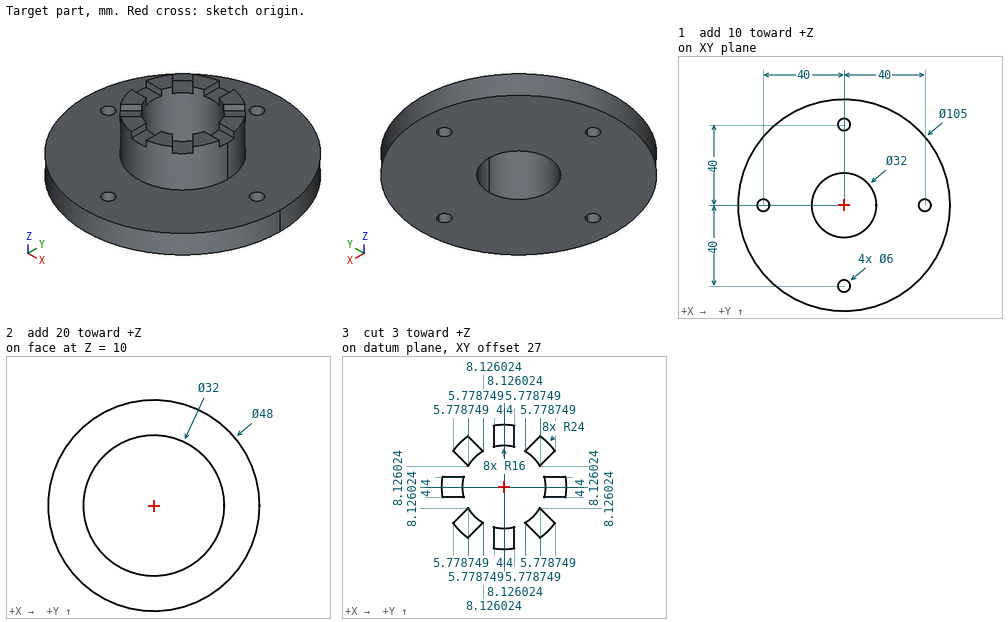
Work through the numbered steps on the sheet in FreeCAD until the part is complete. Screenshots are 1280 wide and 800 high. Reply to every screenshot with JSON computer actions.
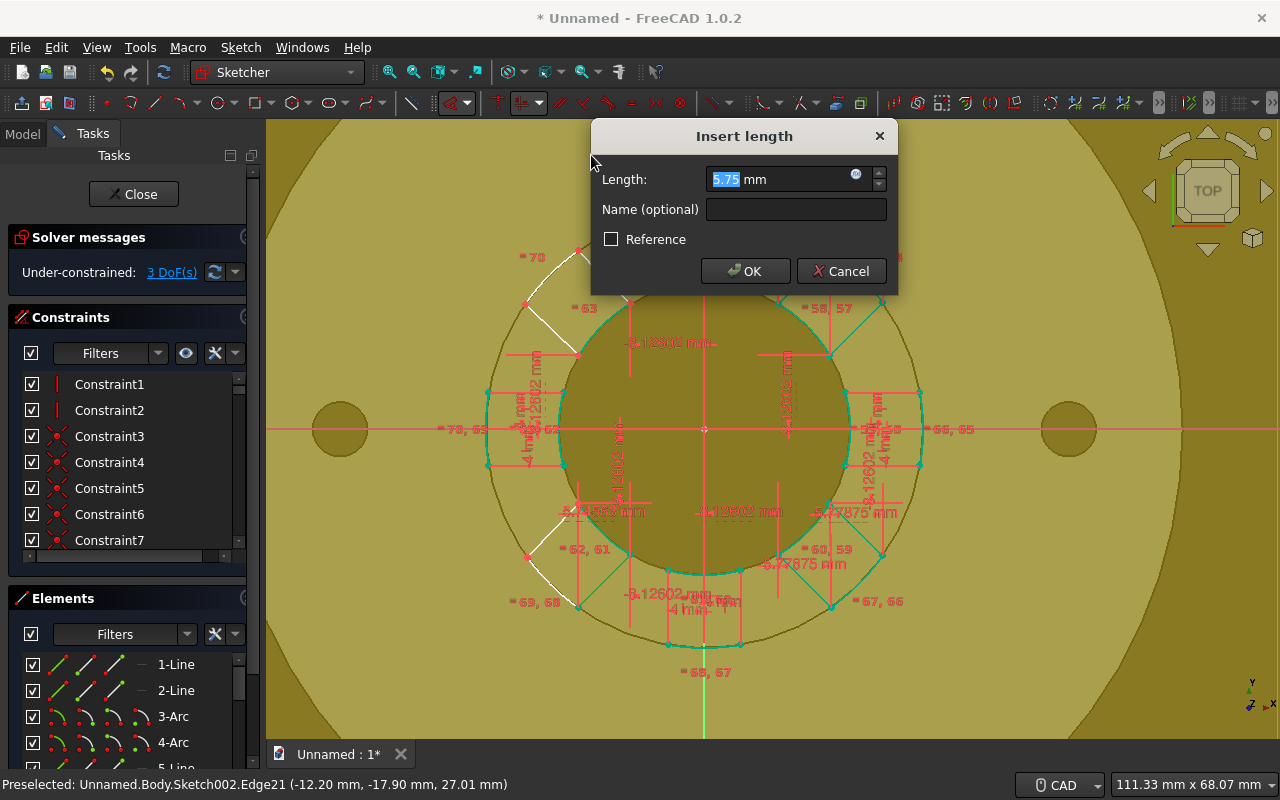
{"action": "type", "text": "5.778749"}
{"action": "key", "text": "Return"}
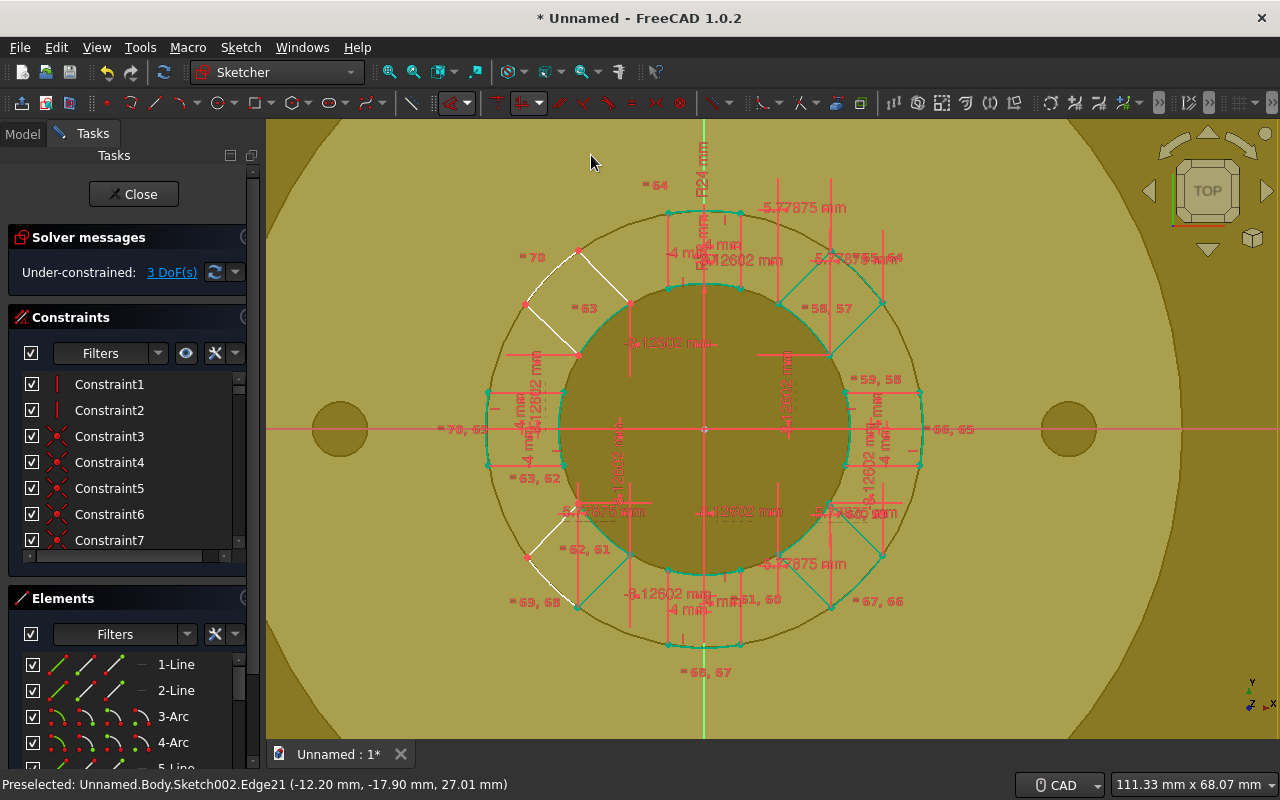
{"action": "left_click", "coordinate": [543, 541]}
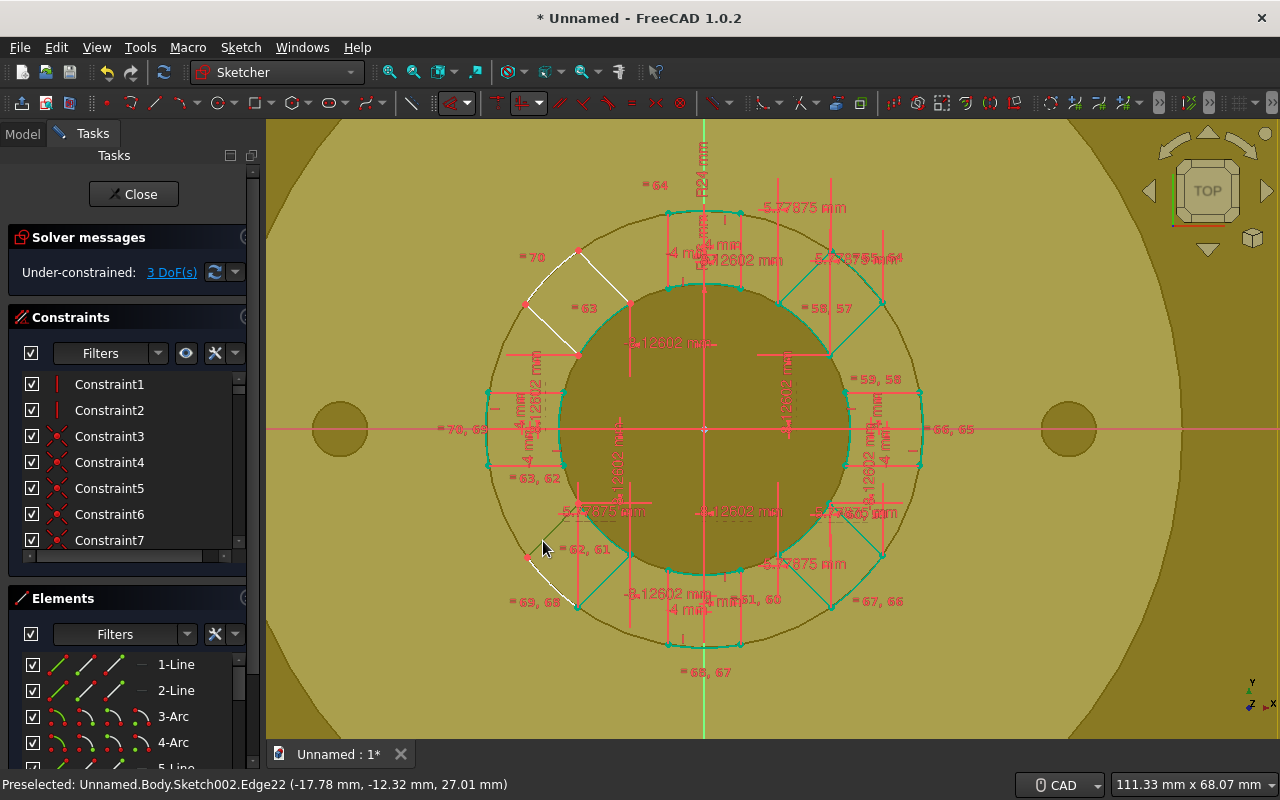
{"action": "left_click", "coordinate": [470, 104]}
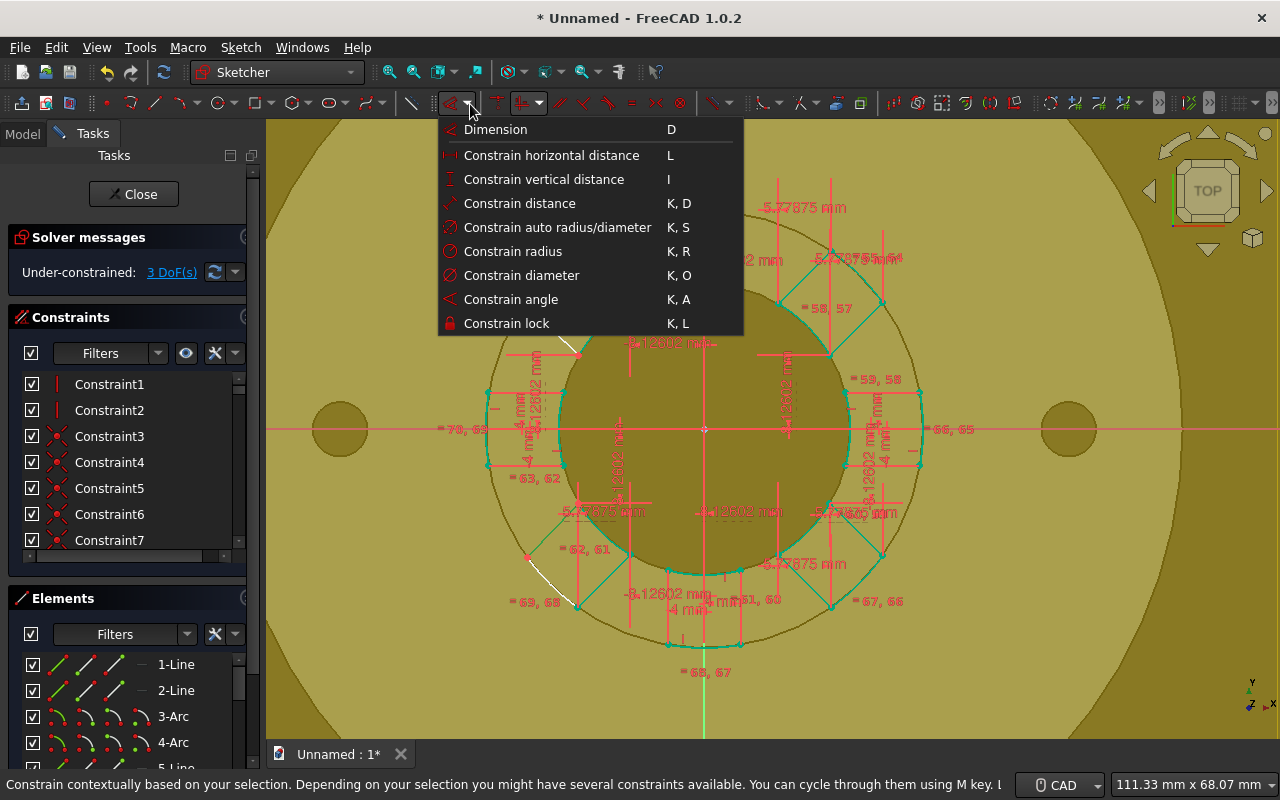
{"action": "left_click", "coordinate": [591, 155]}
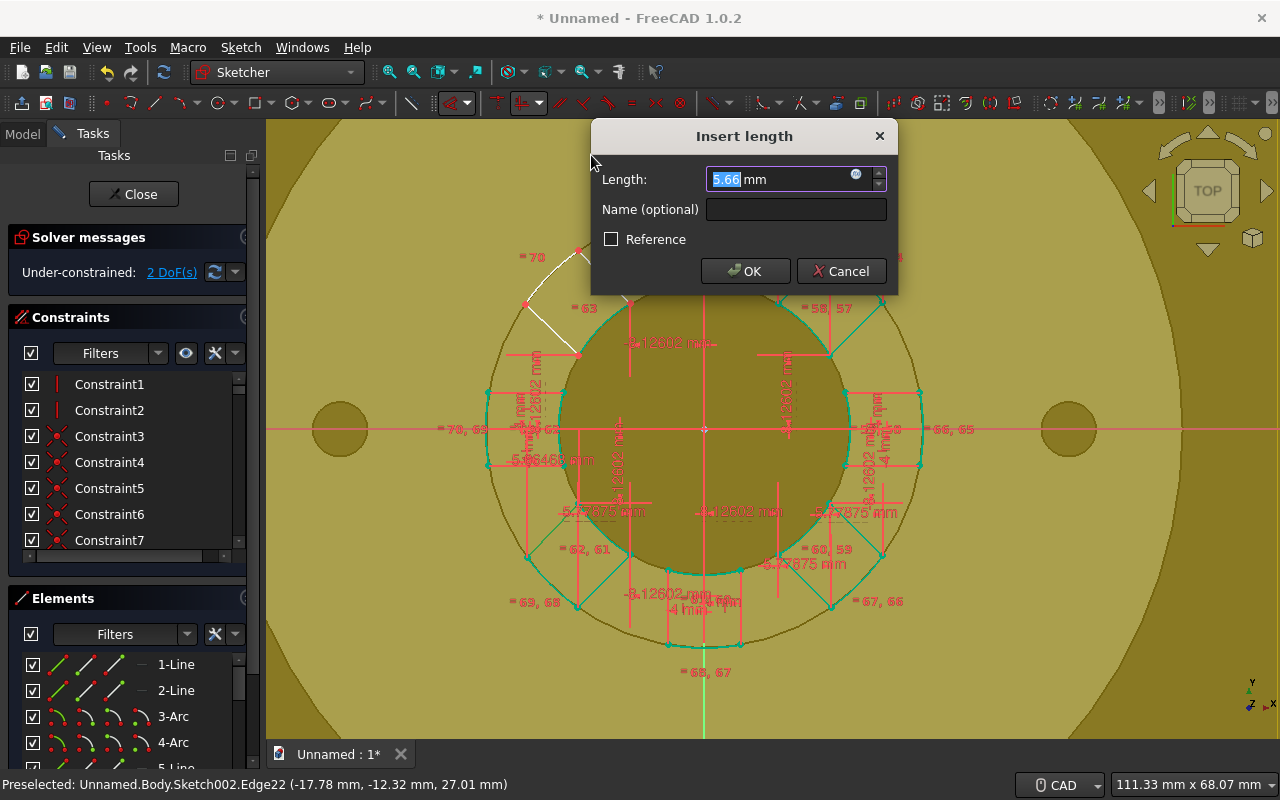
{"action": "type", "text": "5.778749"}
{"action": "key", "text": "Return"}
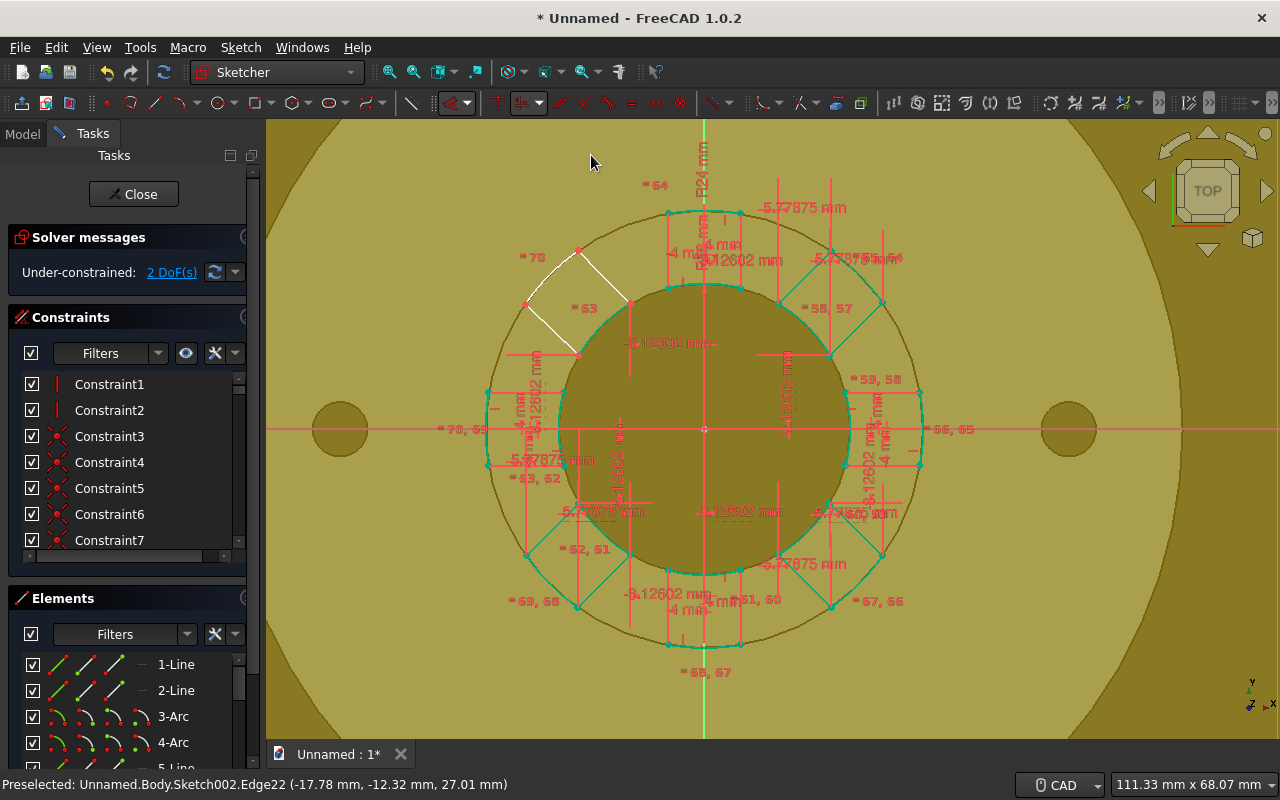
{"action": "left_click", "coordinate": [541, 319]}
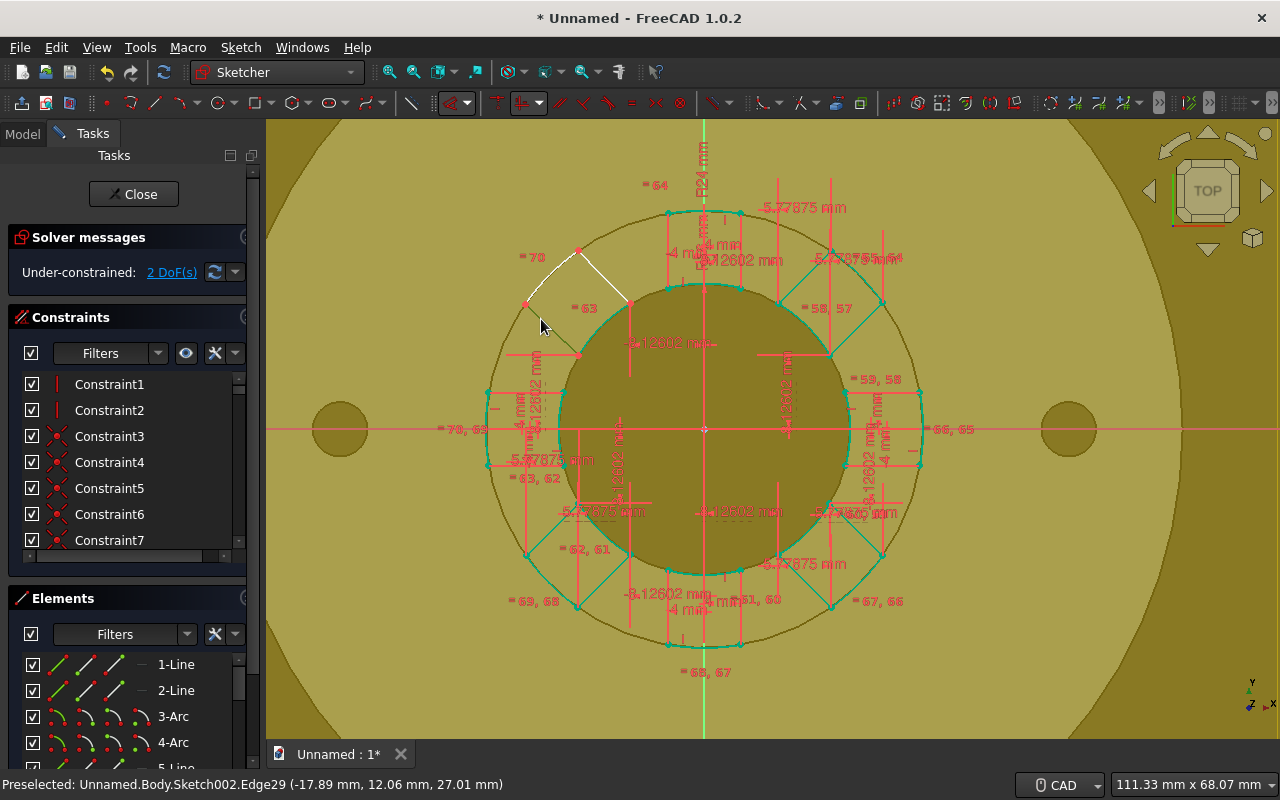
{"action": "left_click", "coordinate": [470, 104]}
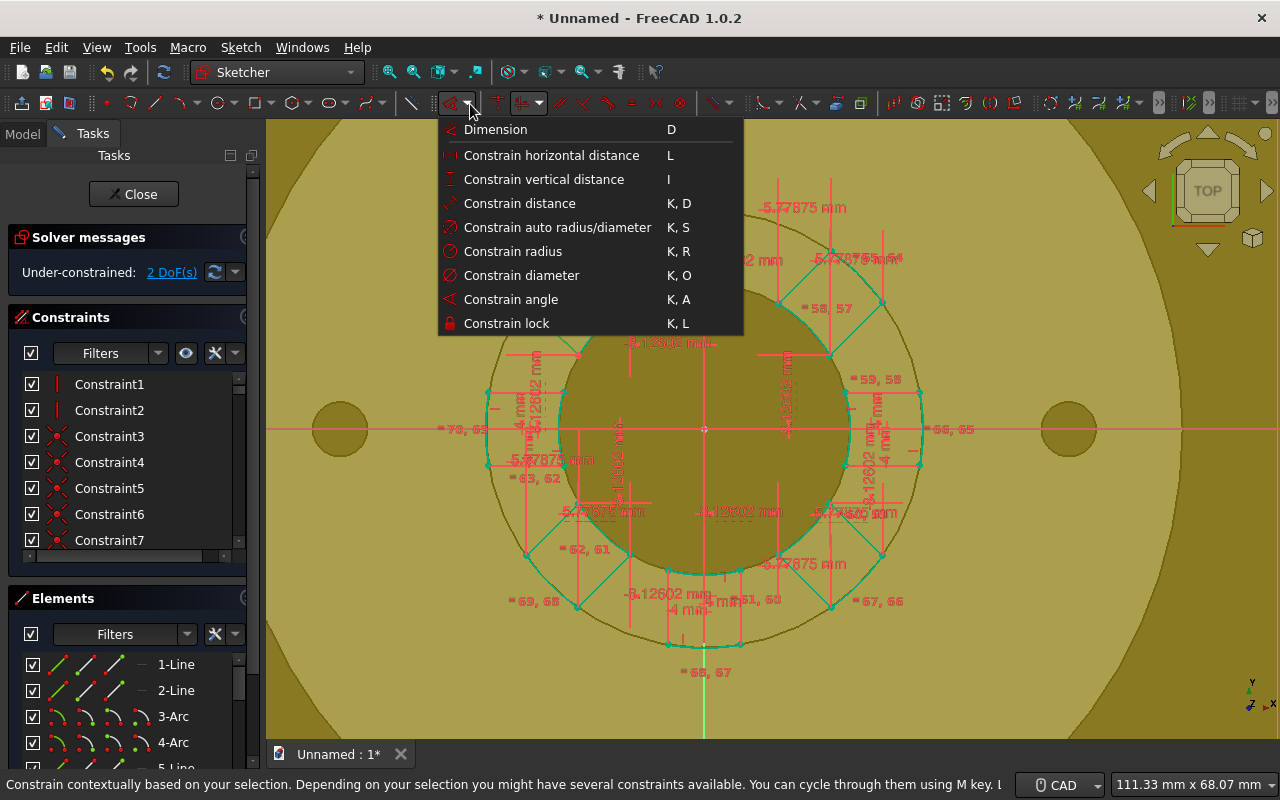
{"action": "left_click", "coordinate": [591, 155]}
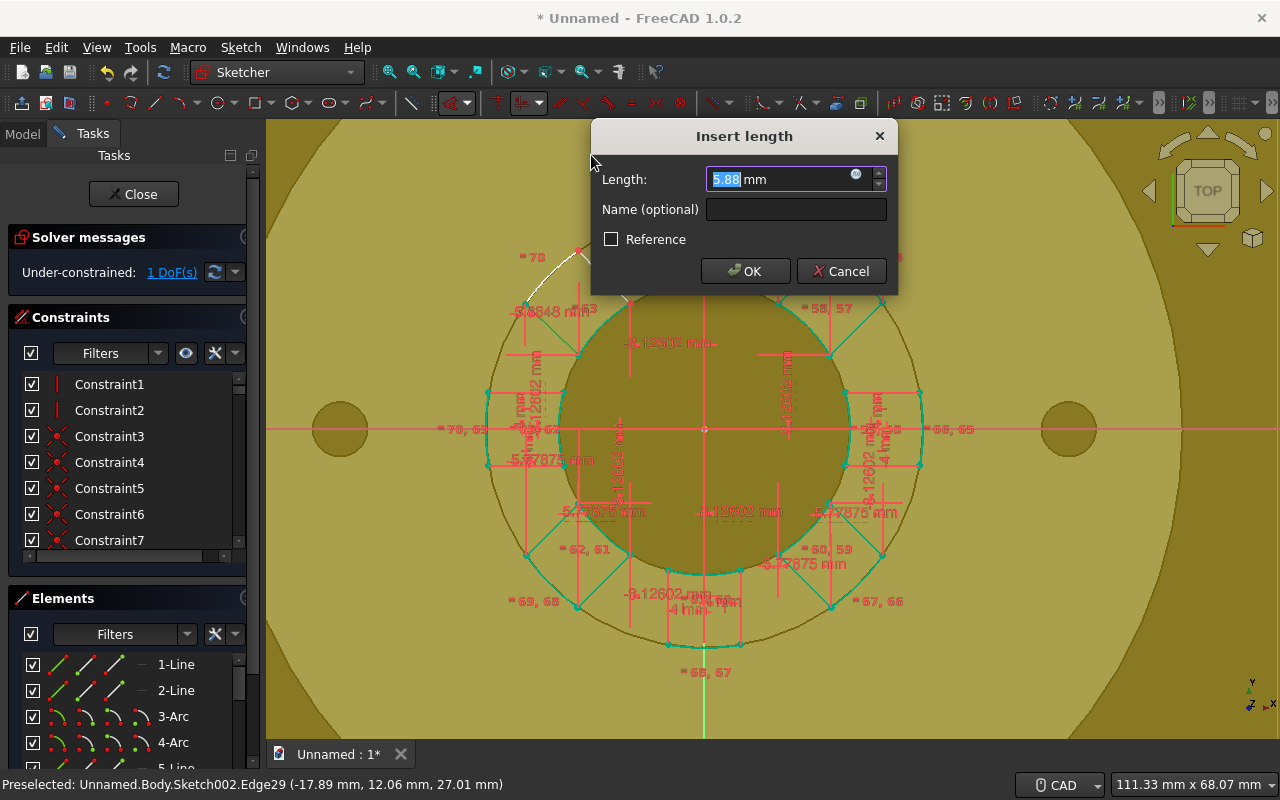
{"action": "type", "text": "5.778749"}
{"action": "key", "text": "Return"}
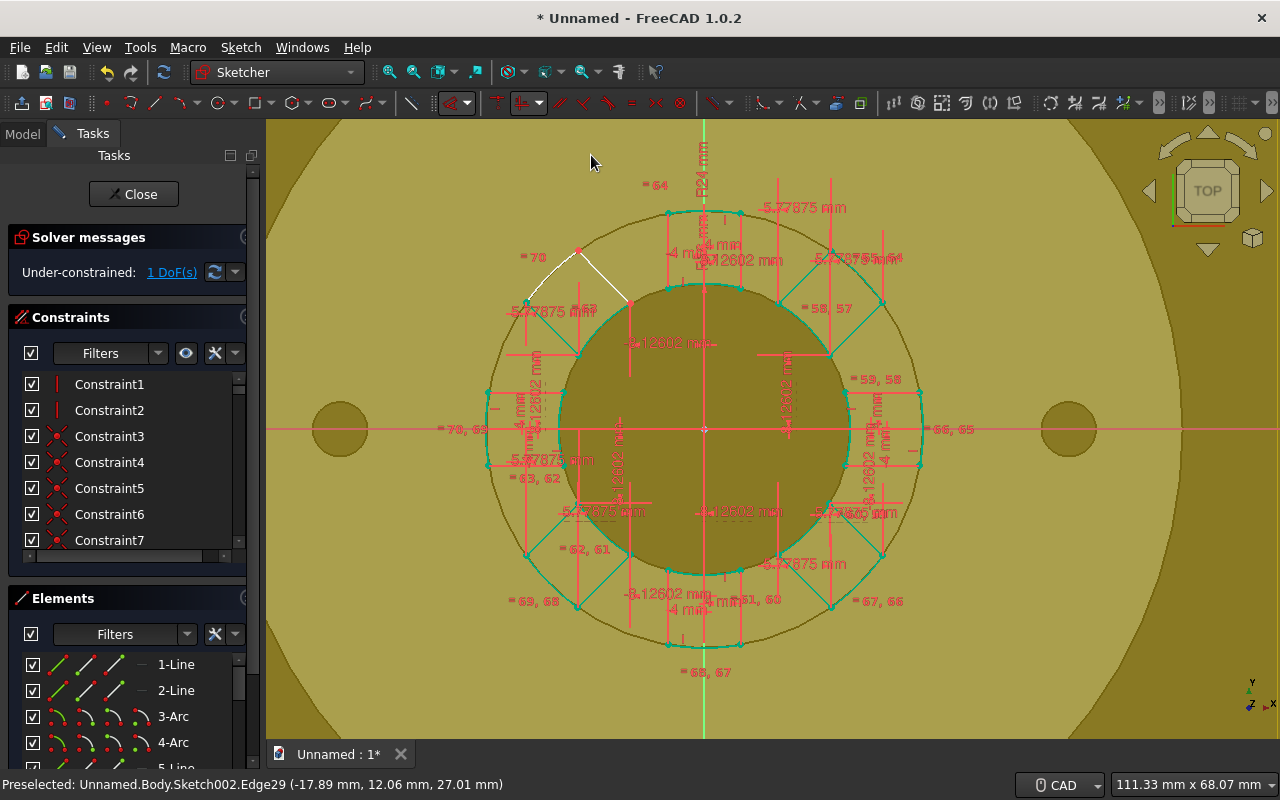
{"action": "left_click", "coordinate": [615, 288]}